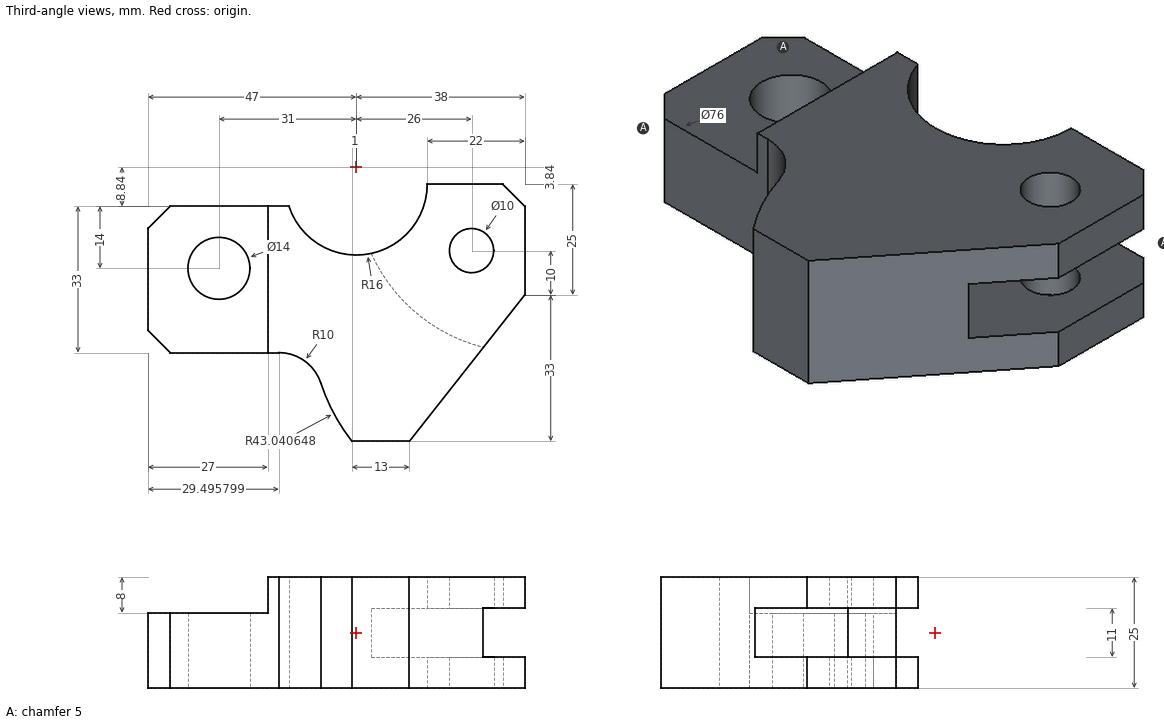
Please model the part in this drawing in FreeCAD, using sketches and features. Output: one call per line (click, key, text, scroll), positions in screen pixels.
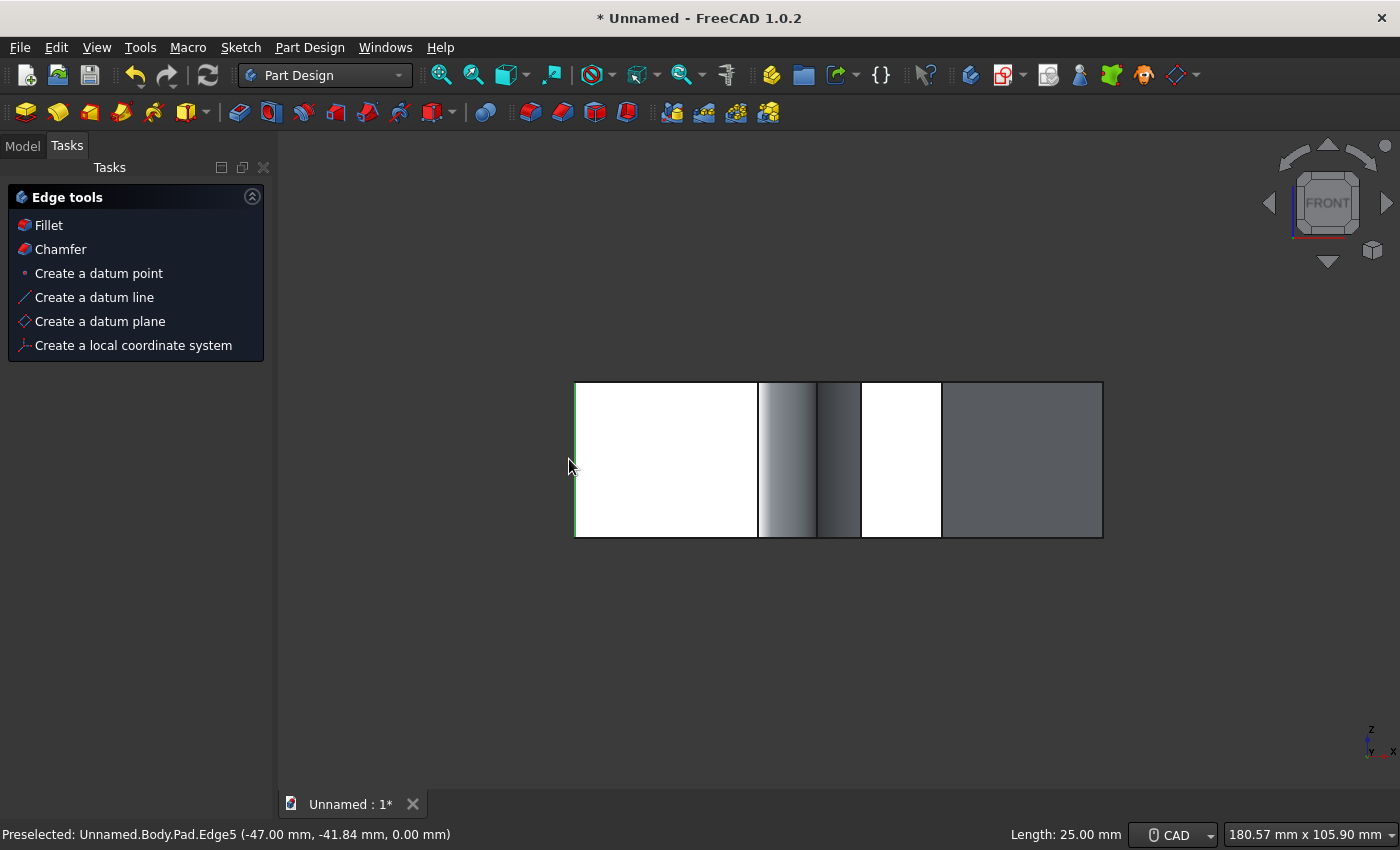
key(3)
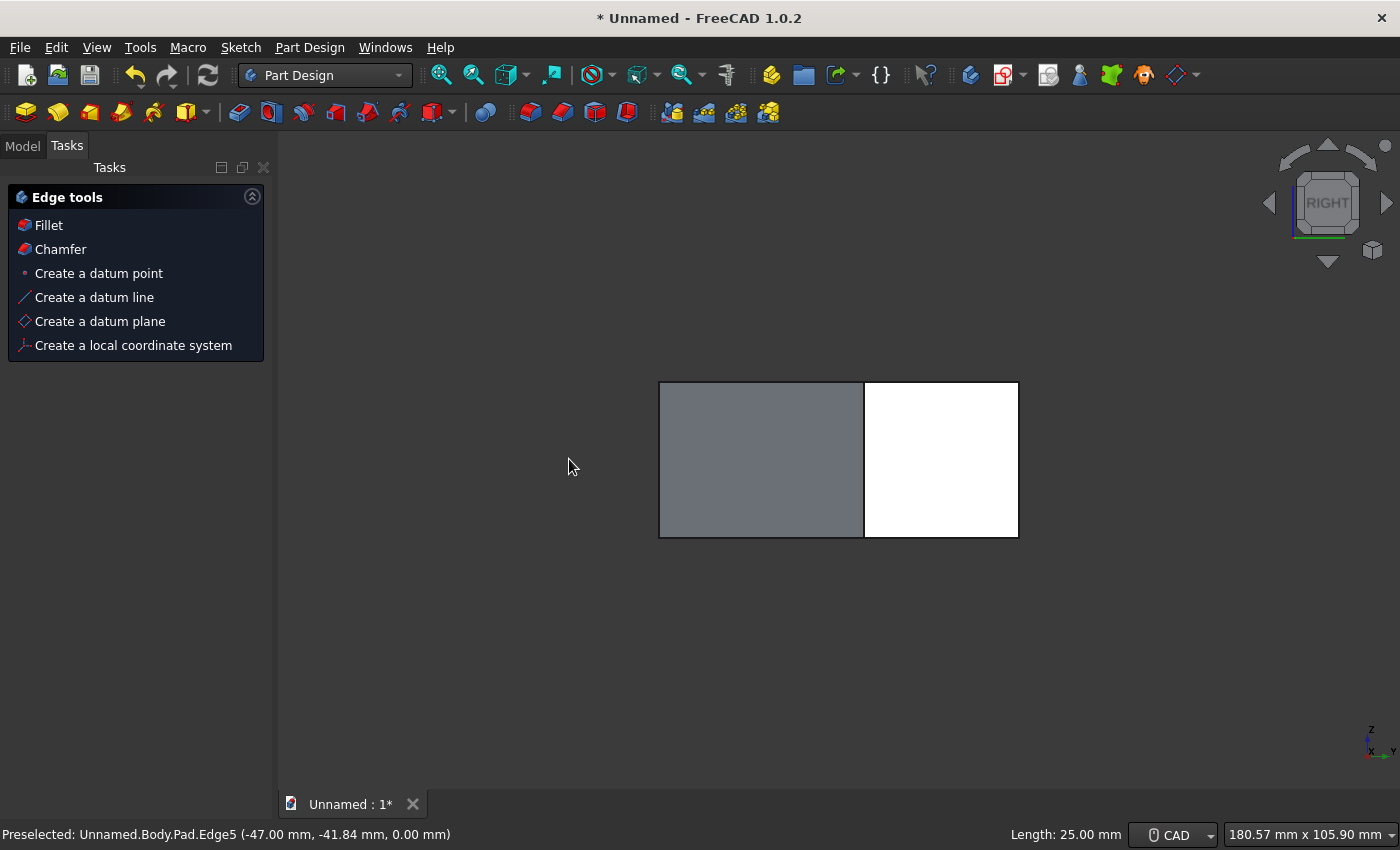
key(v)
key(f)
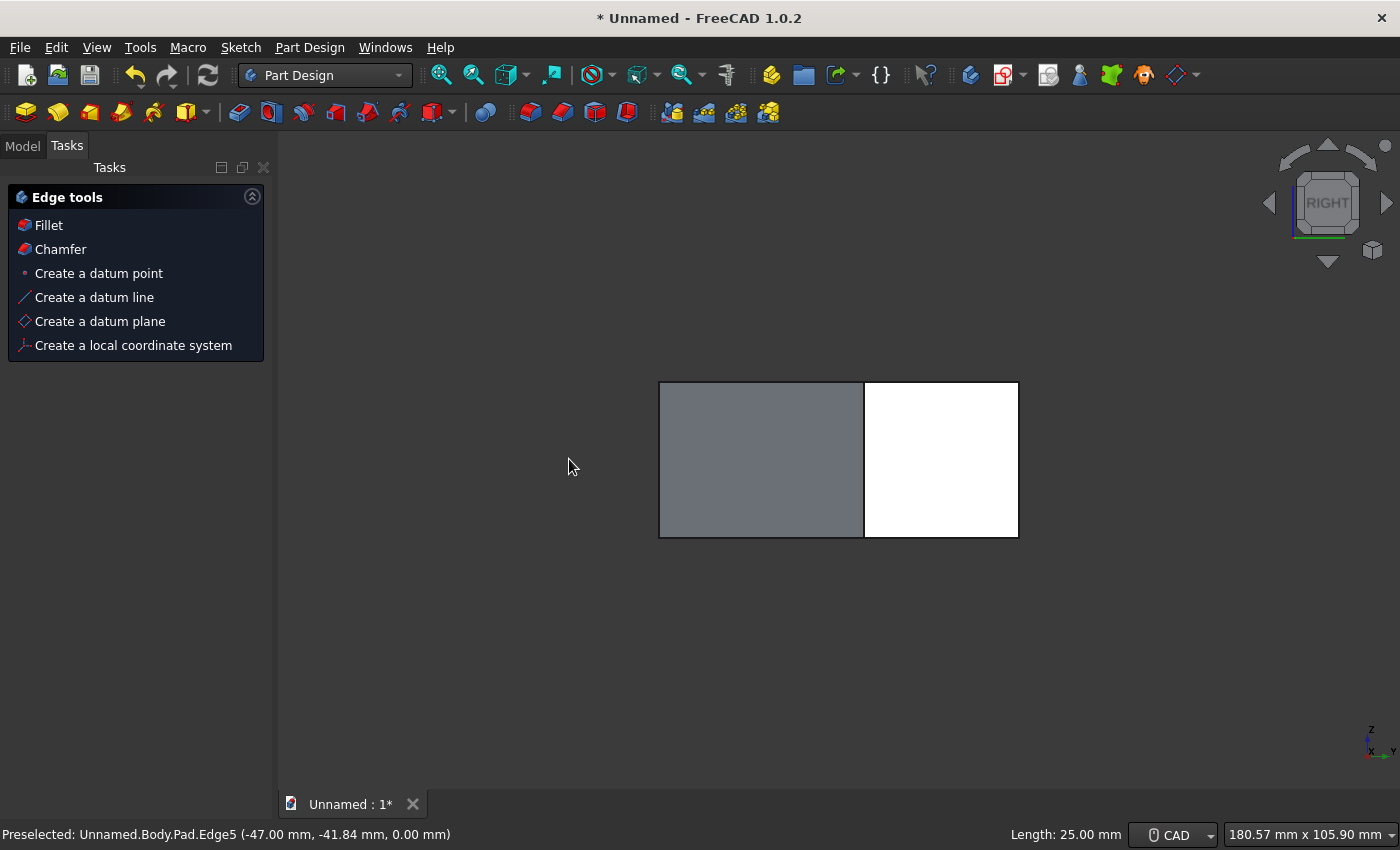
click(1019, 459, ctrl)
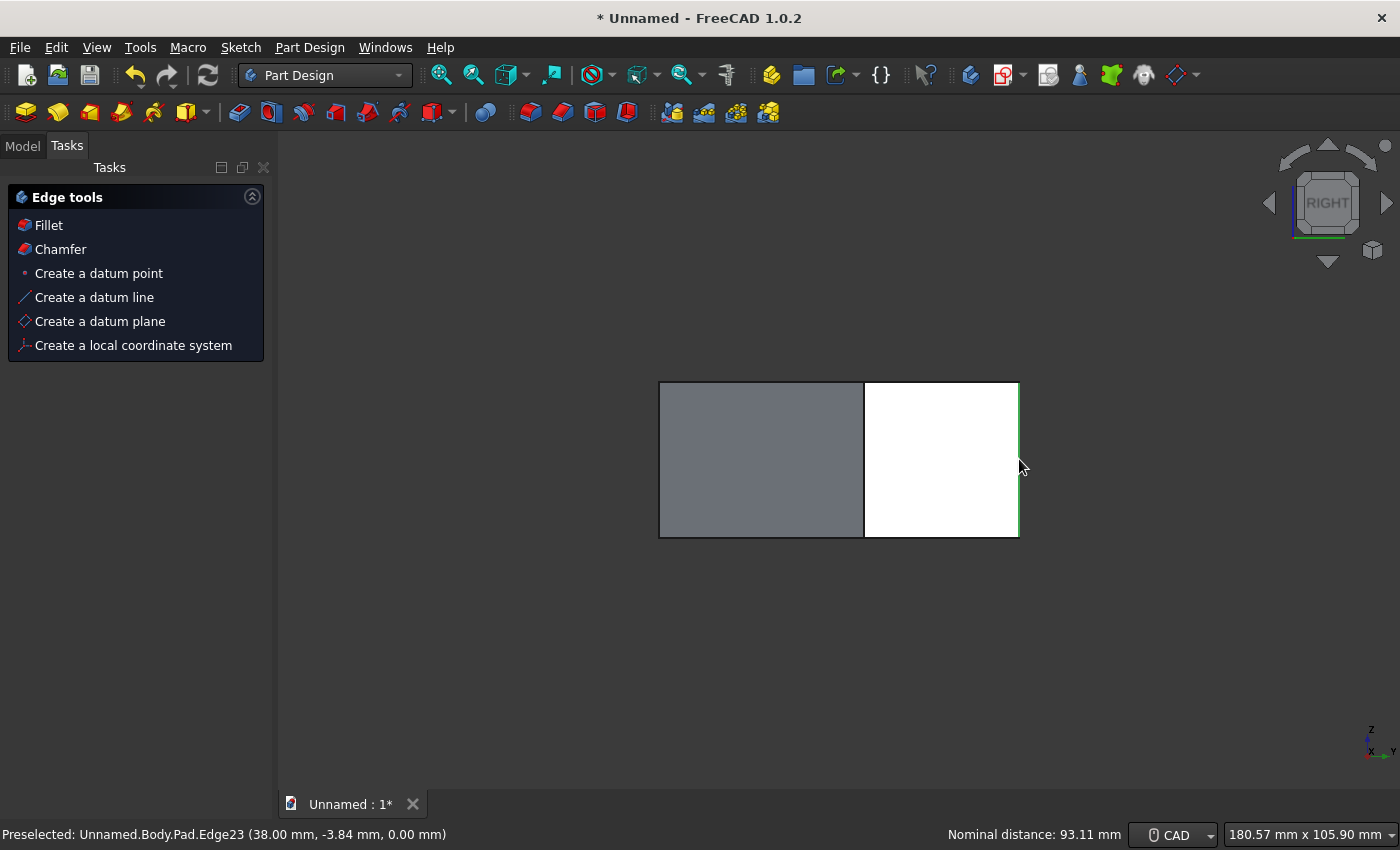
key(5)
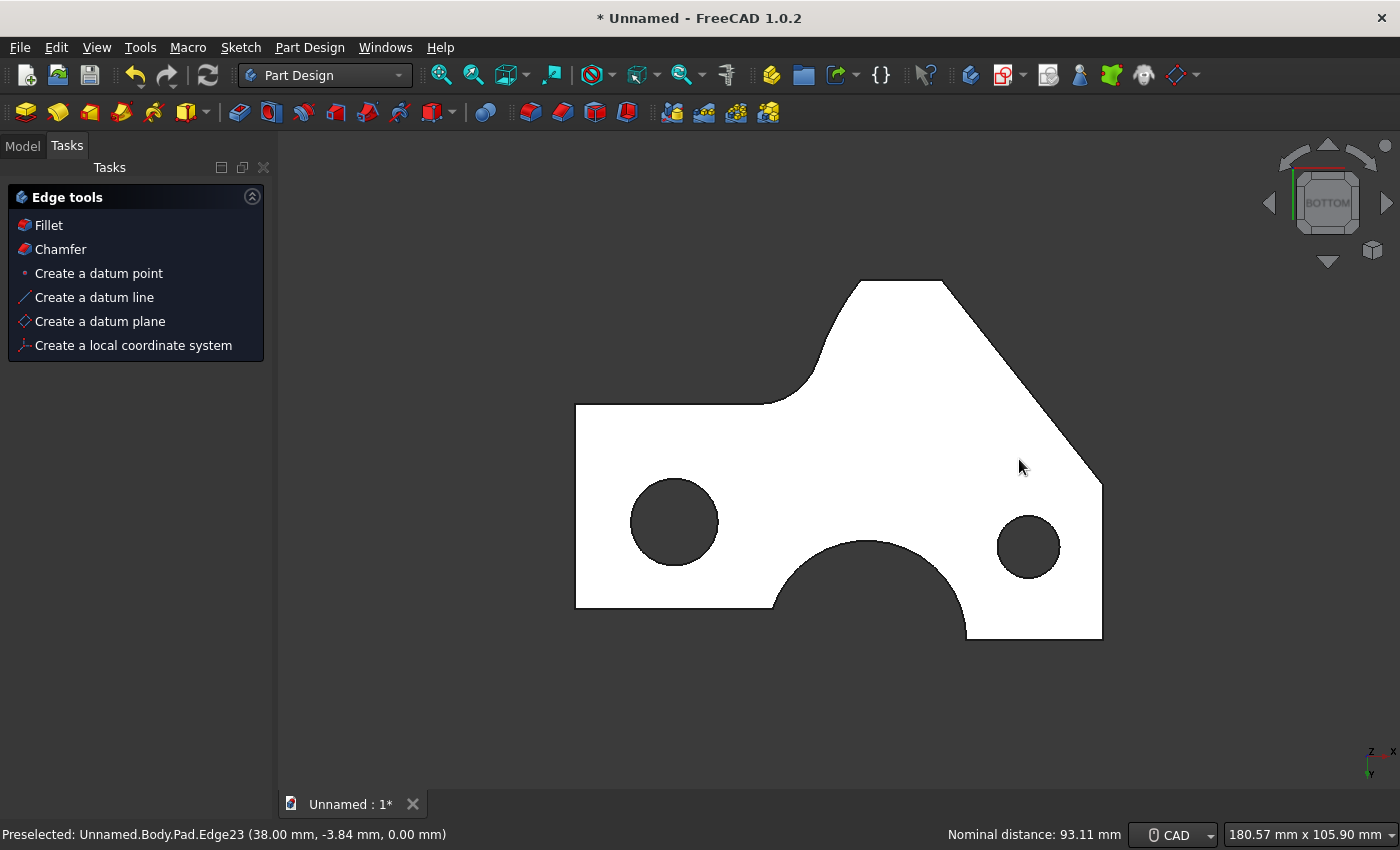
key(4)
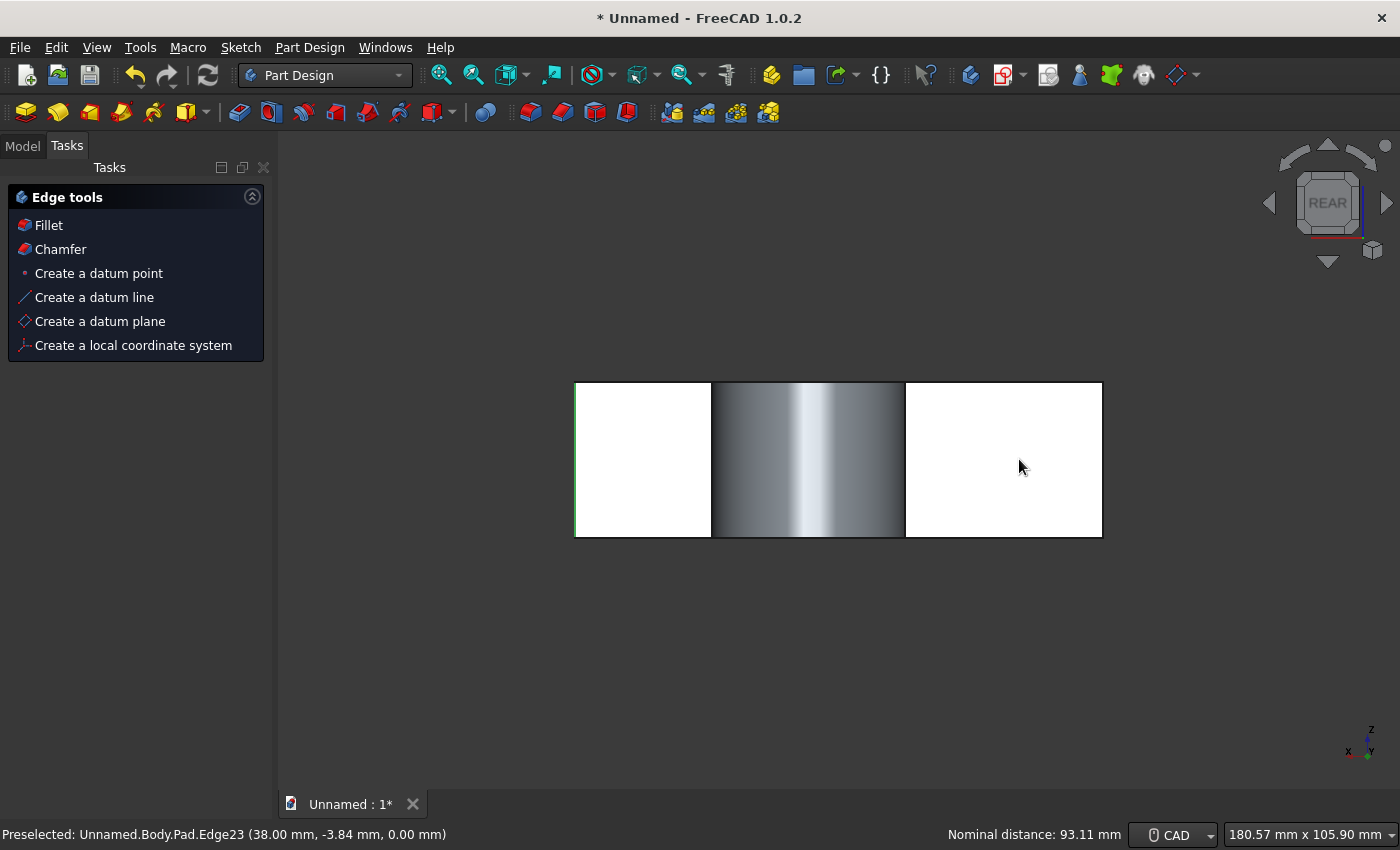
click(1103, 459, ctrl)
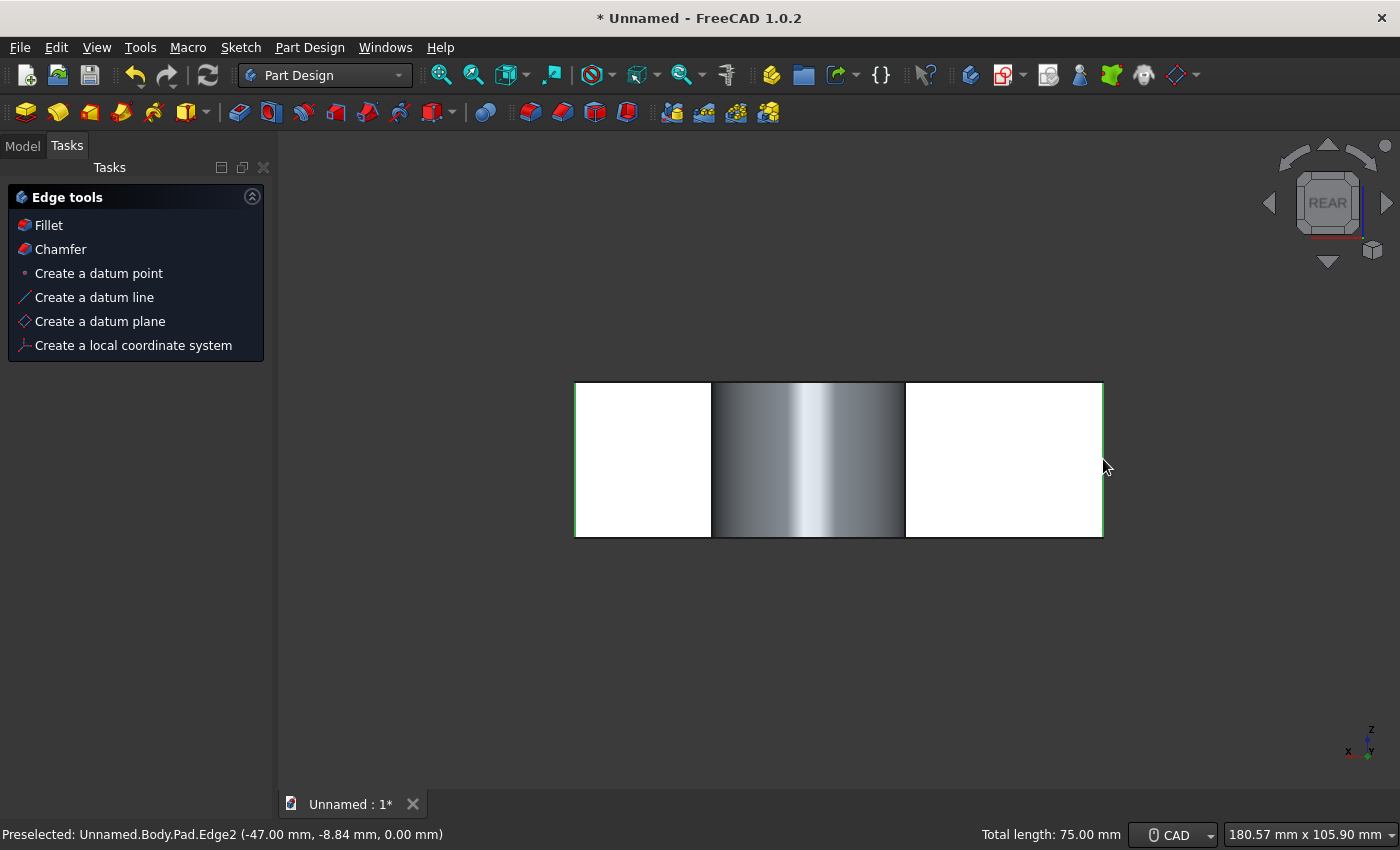
click(564, 112)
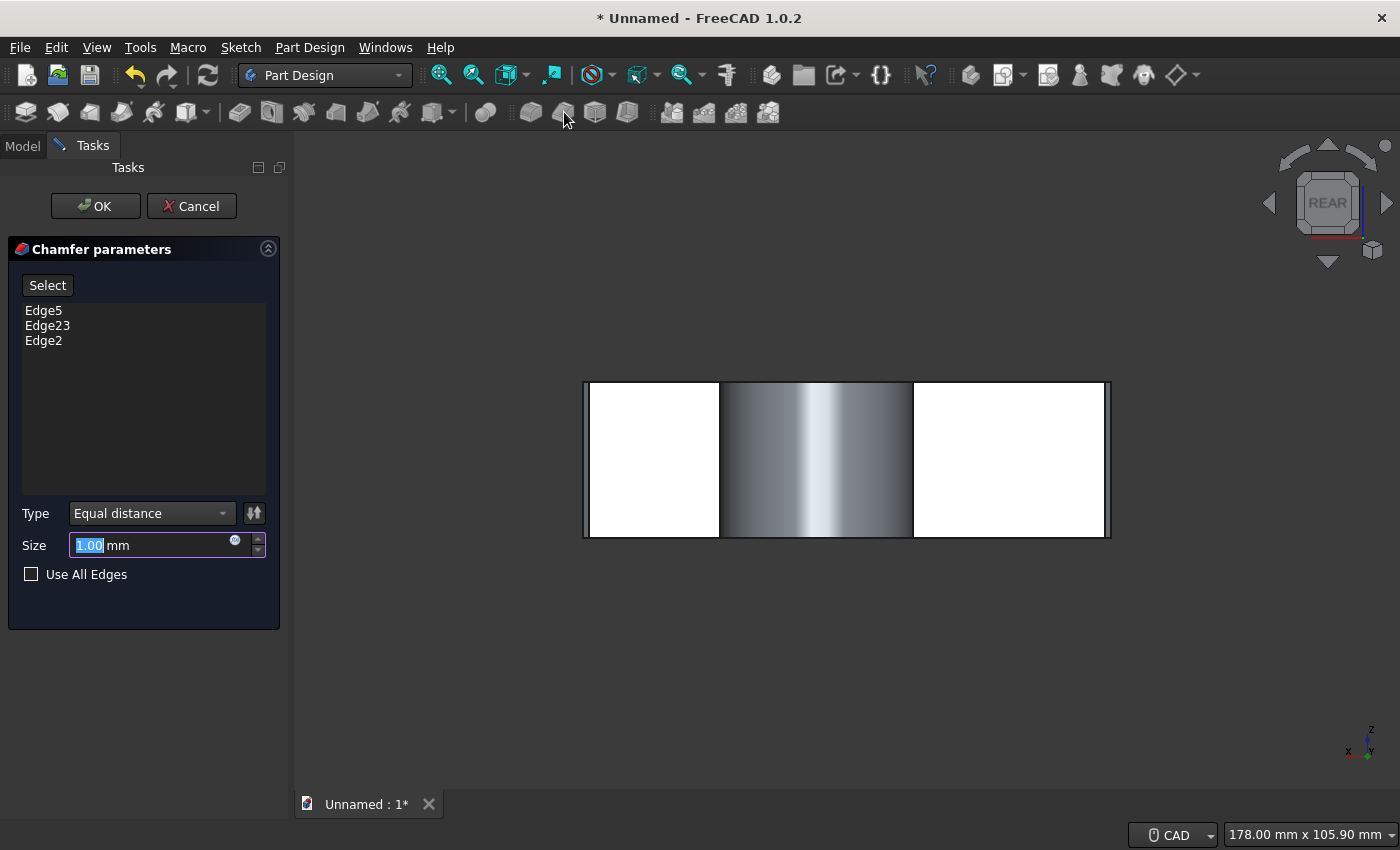
text(5)
key(Tab)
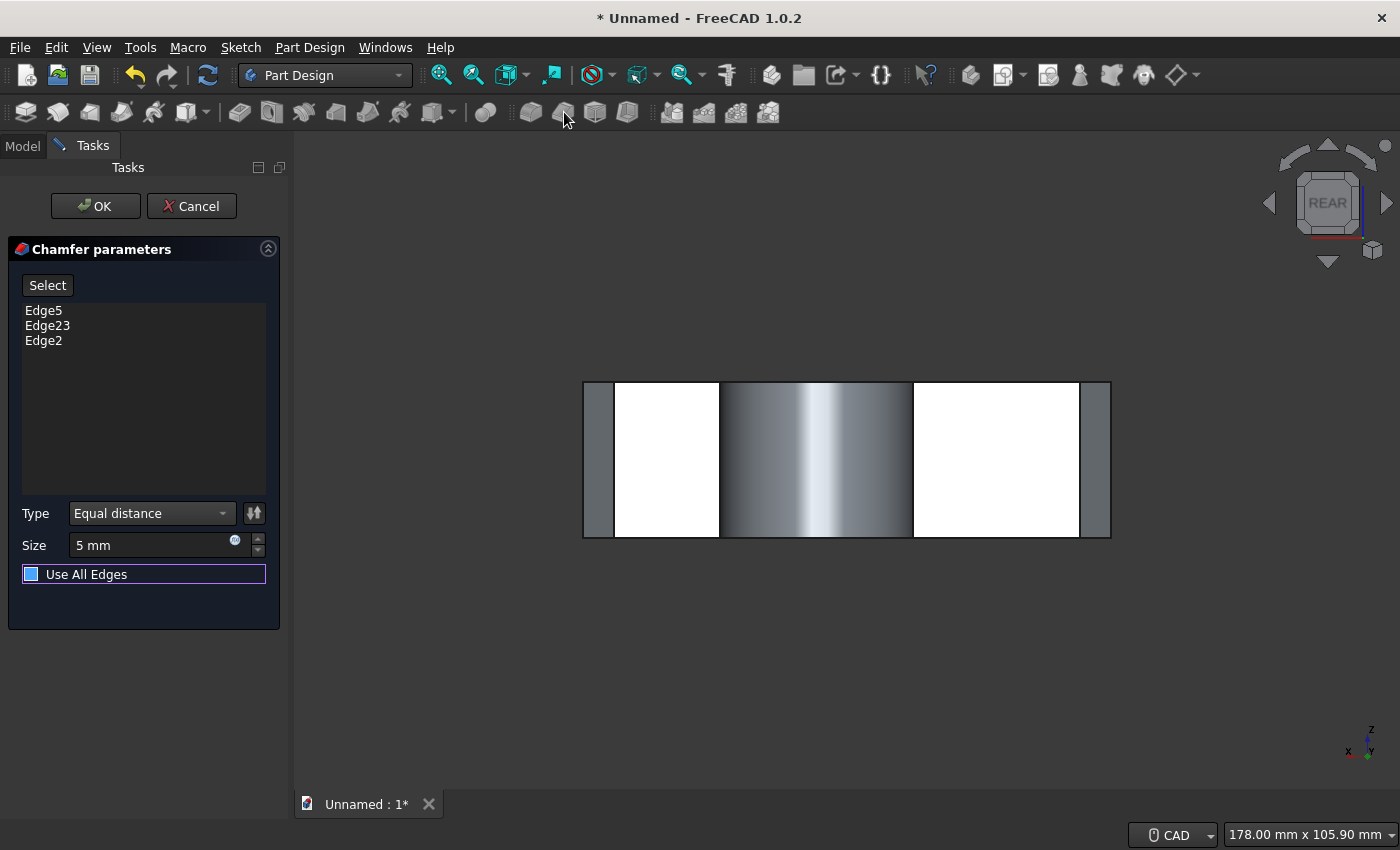
click(96, 206)